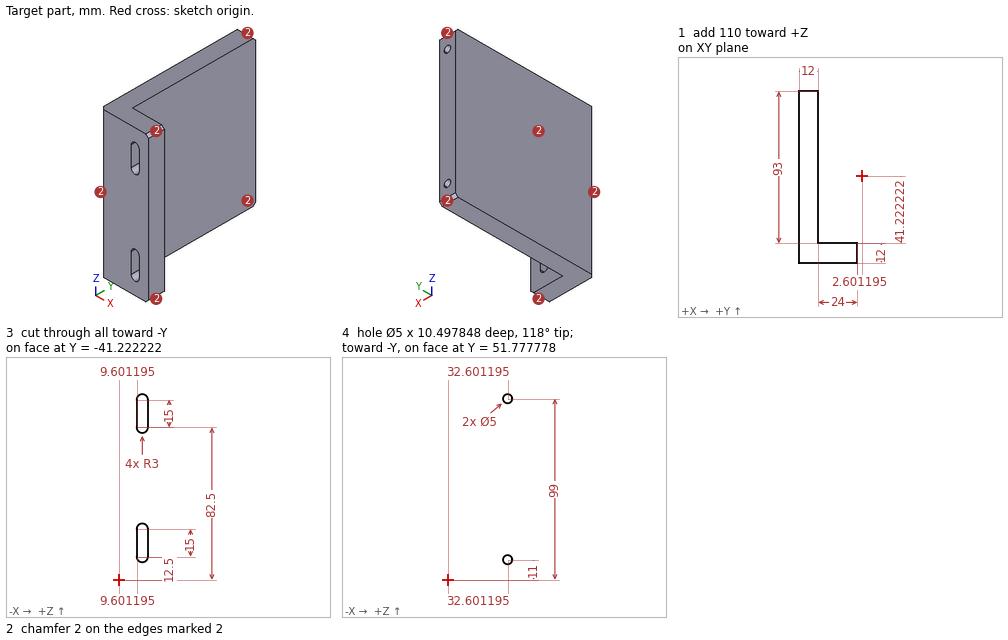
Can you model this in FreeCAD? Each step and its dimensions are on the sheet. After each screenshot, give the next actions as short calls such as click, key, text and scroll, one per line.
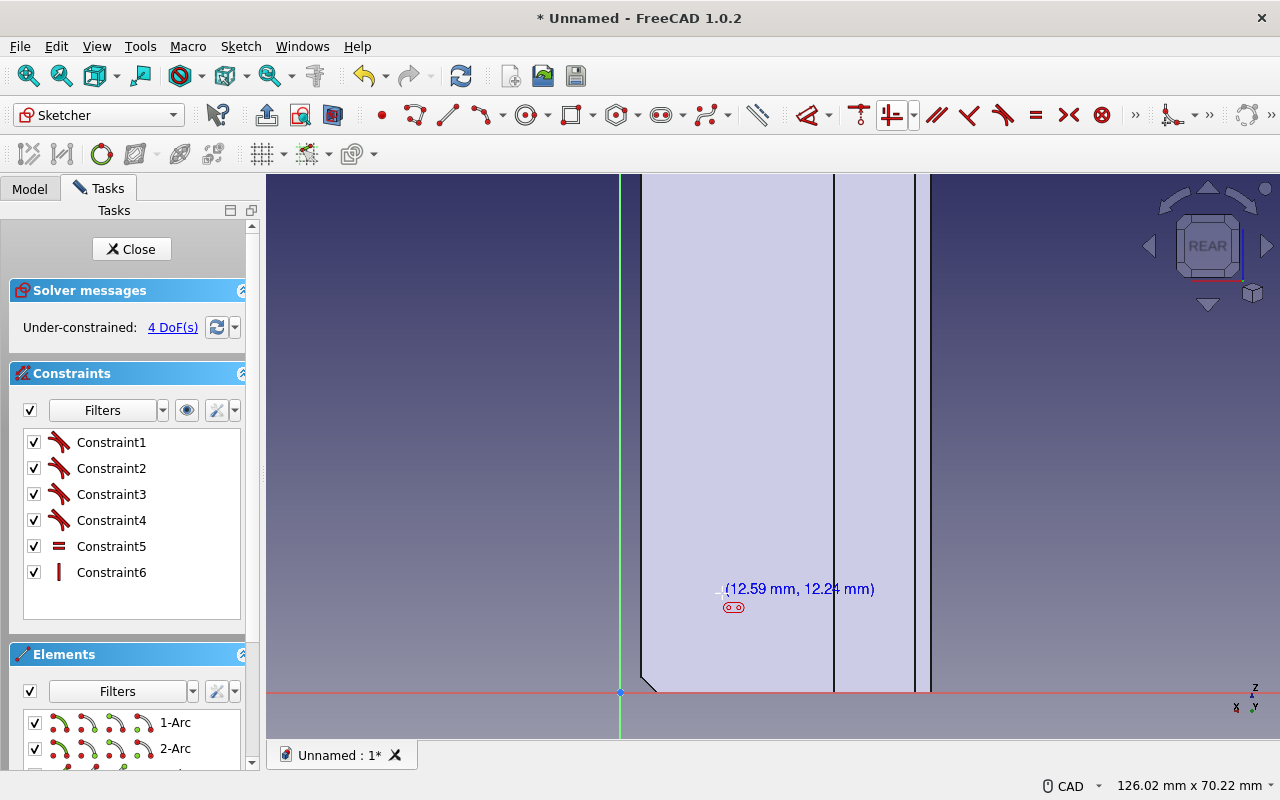
click(722, 592)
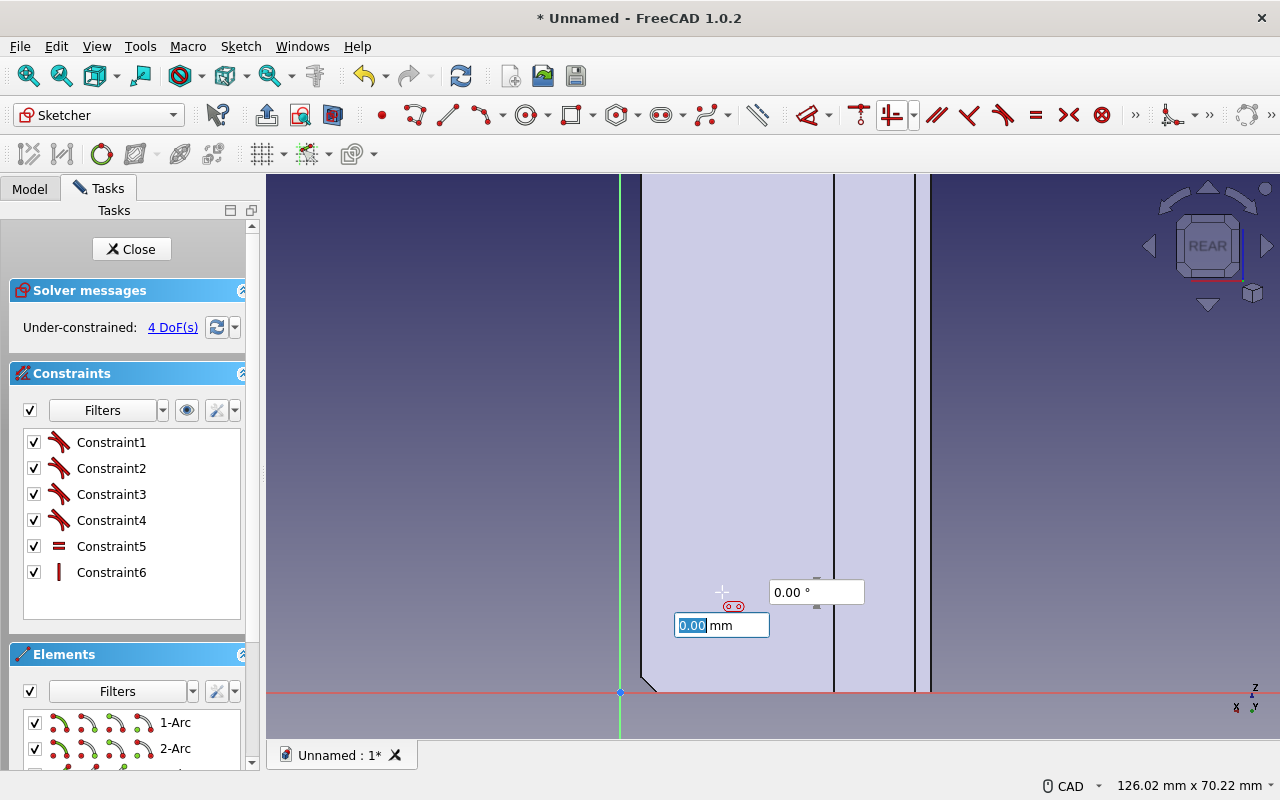
click(722, 472)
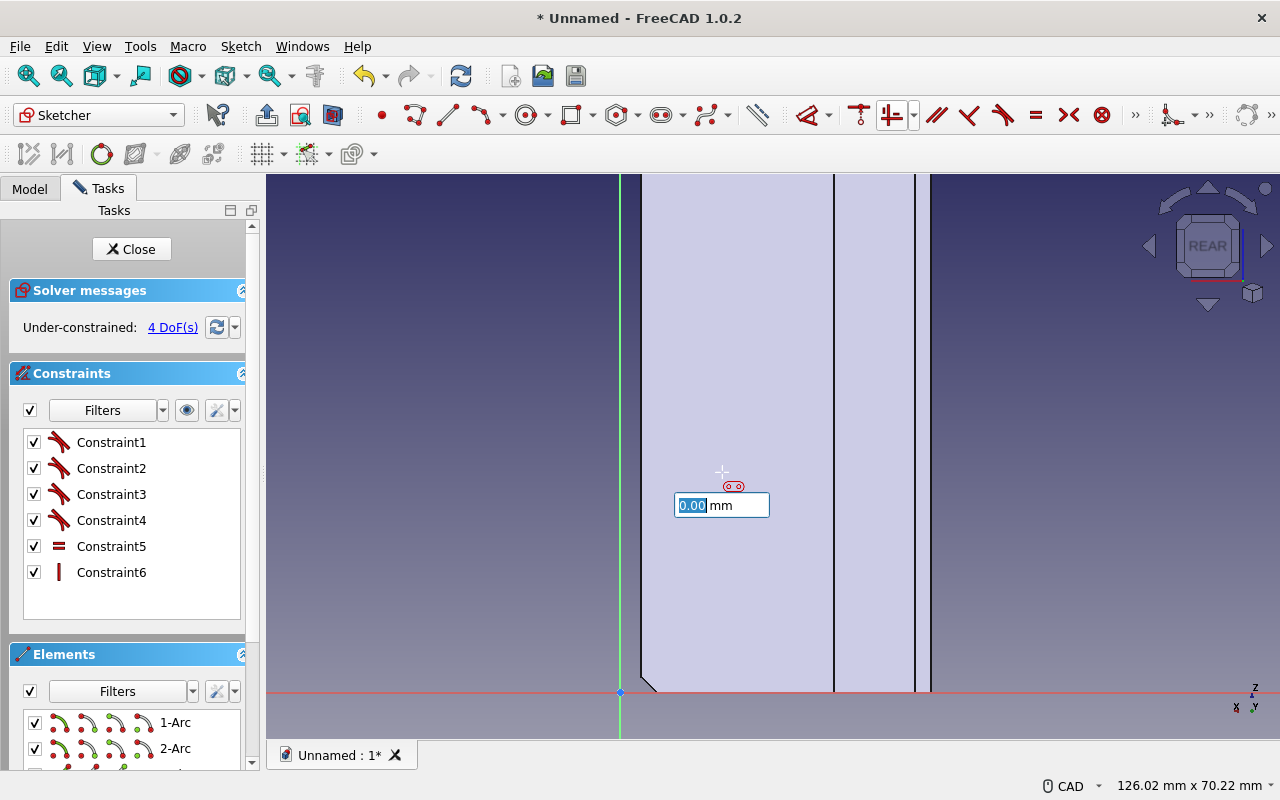
click(746, 532)
key(Escape)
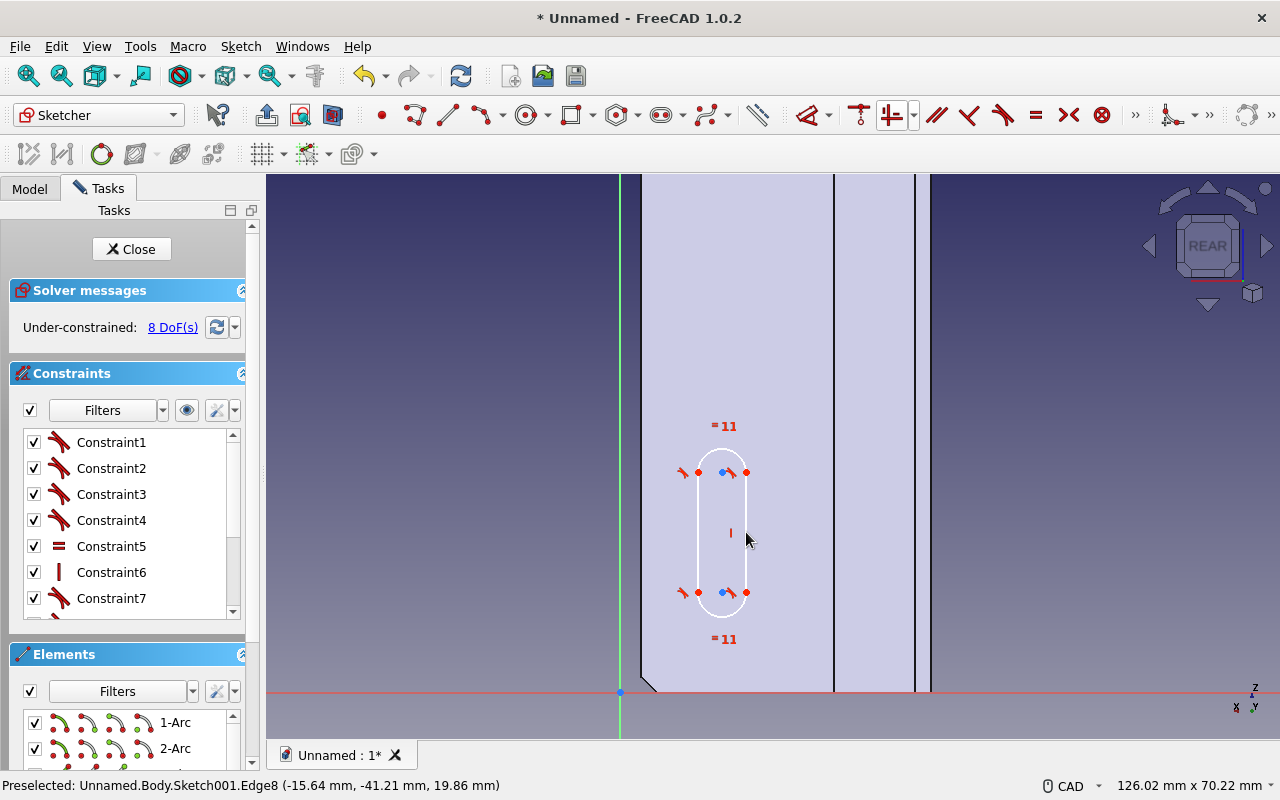
scroll(722, 594, down, 4)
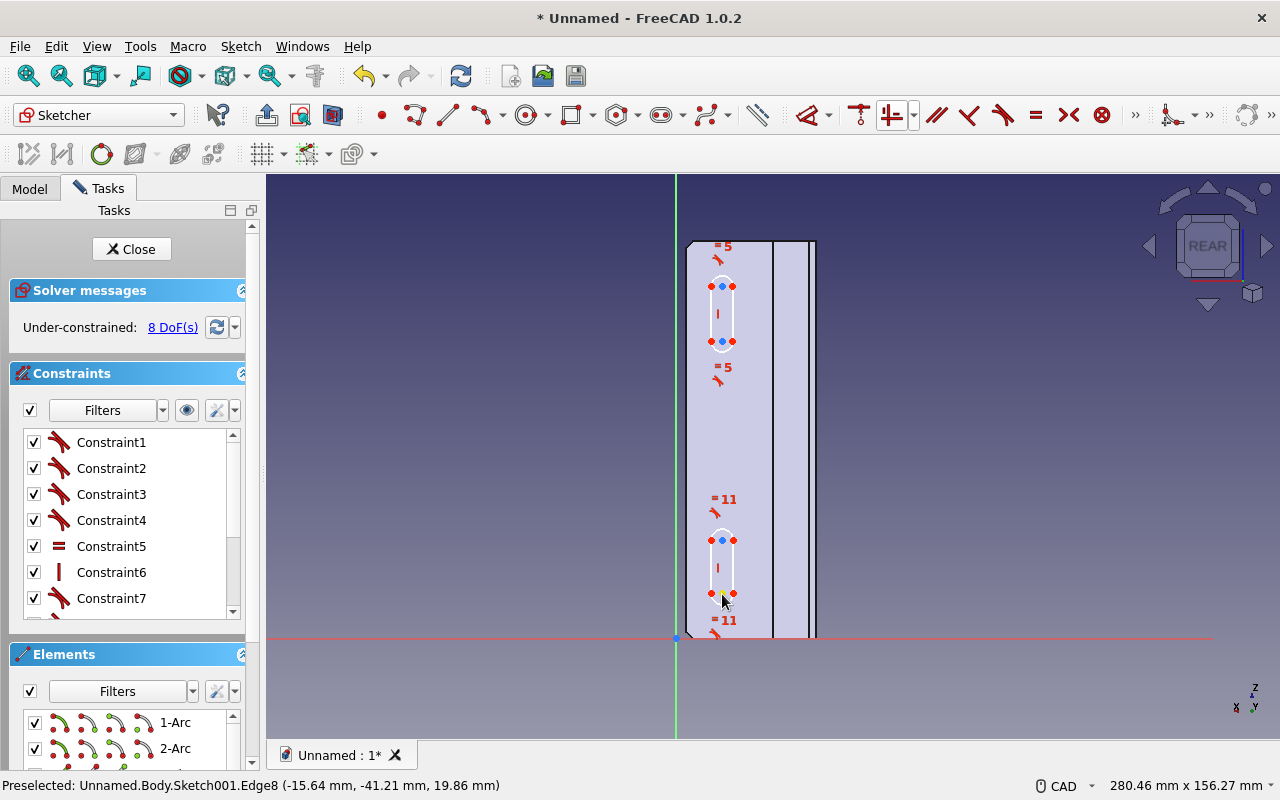
scroll(716, 350, up, 2)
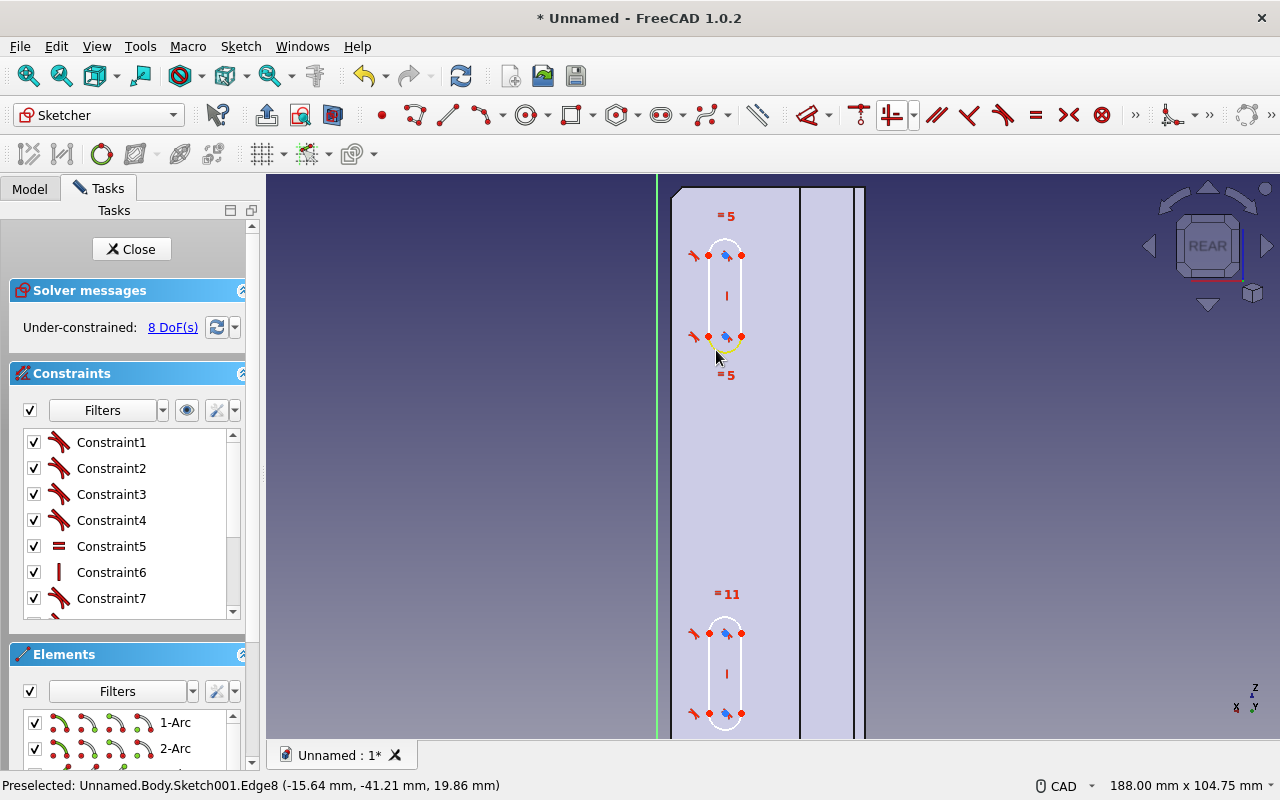
click(716, 350)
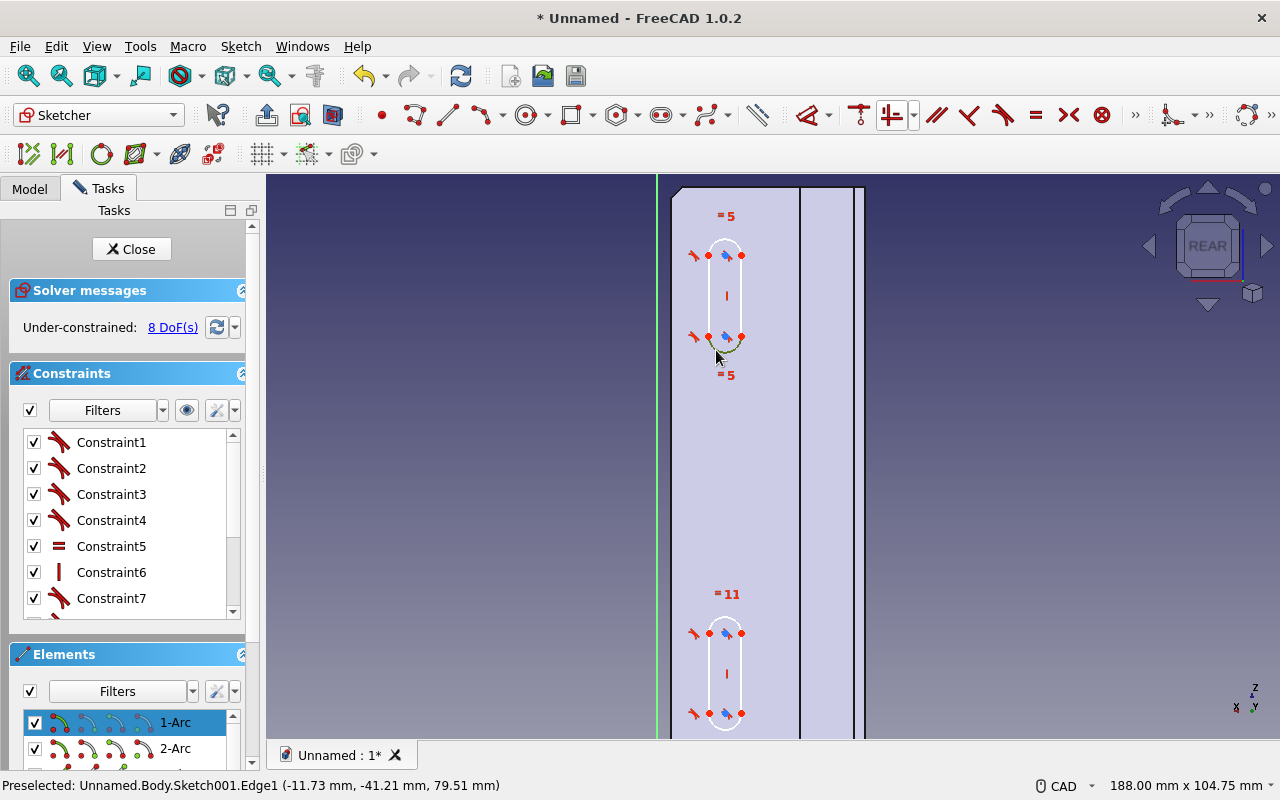
scroll(716, 348, down, 2)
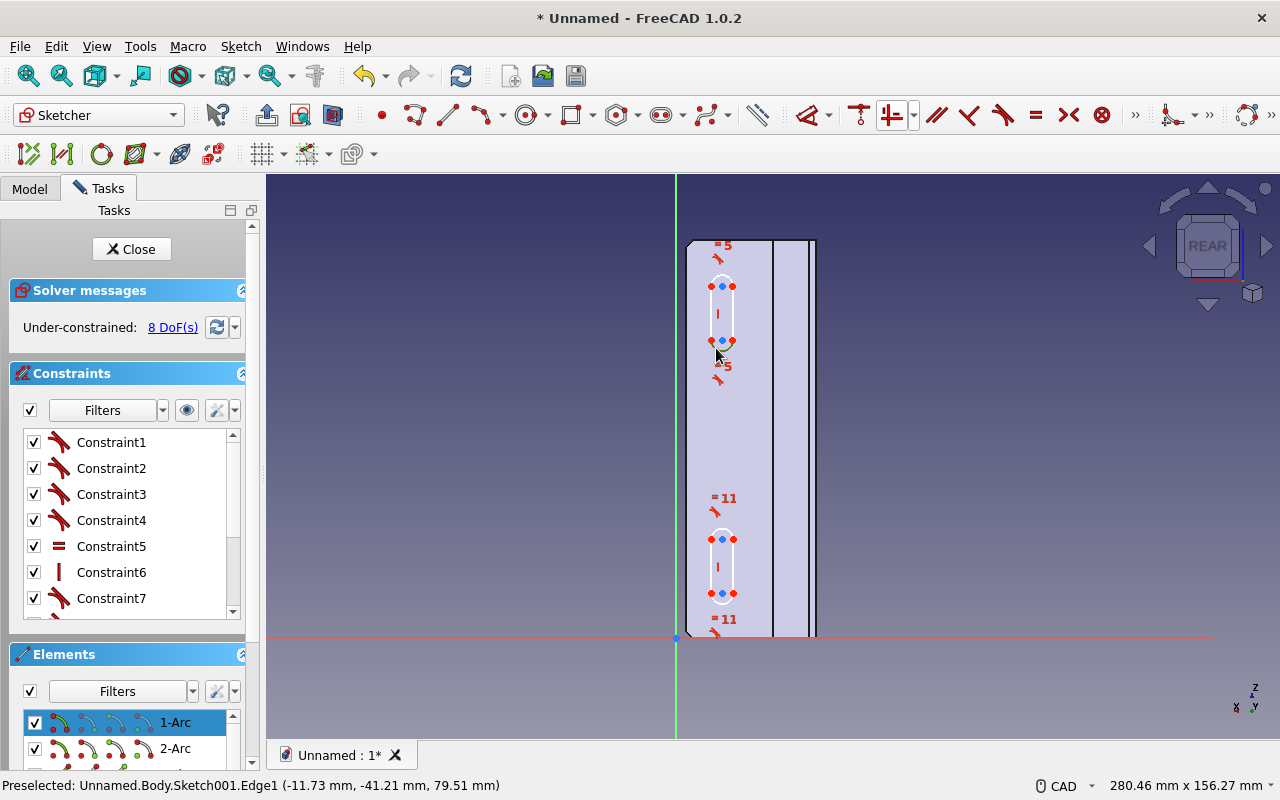
scroll(716, 602, up, 2)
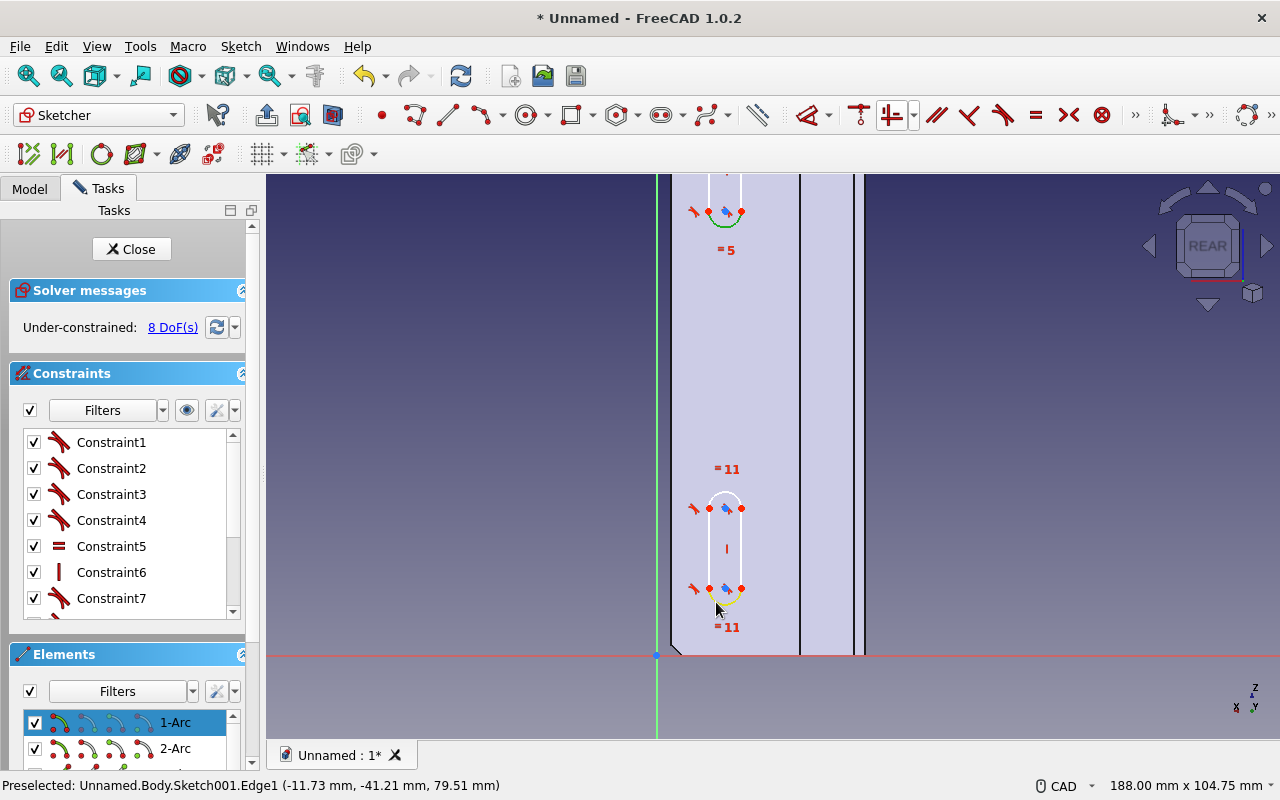
click(716, 602)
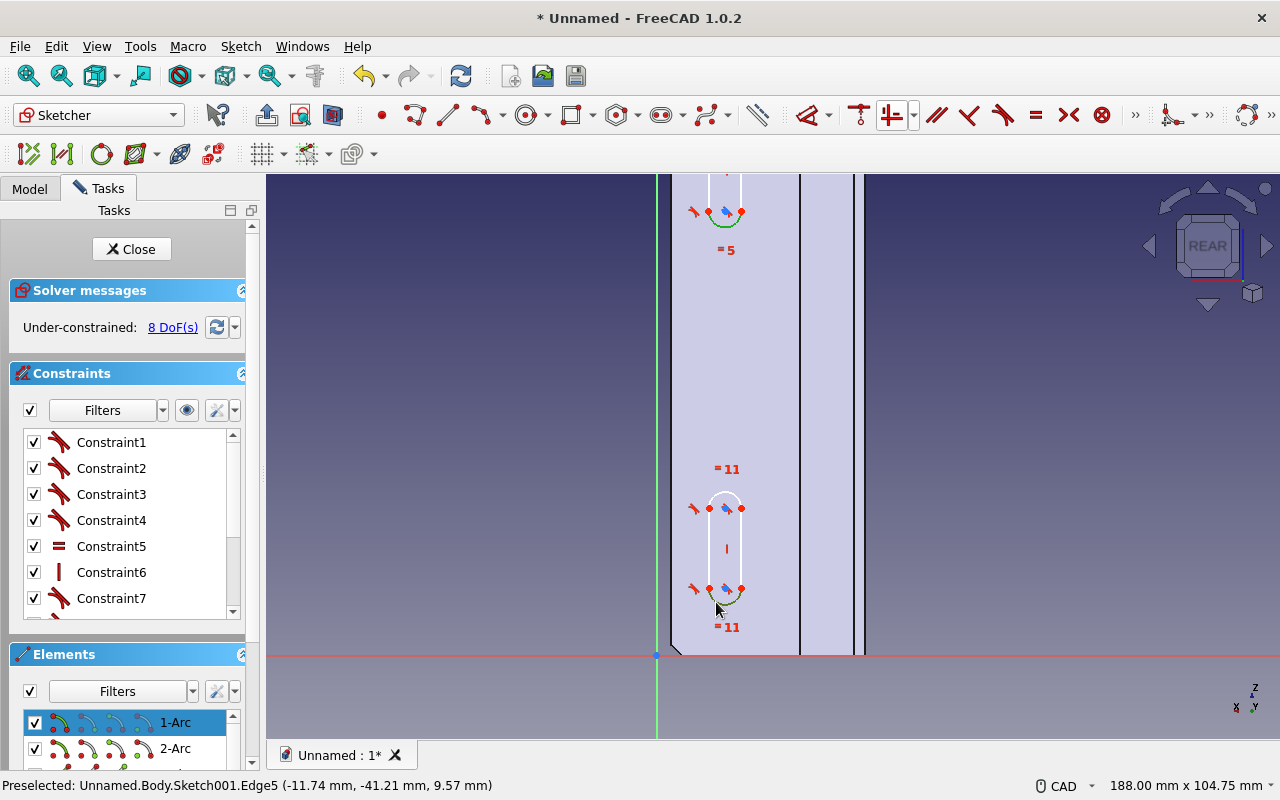
click(1036, 116)